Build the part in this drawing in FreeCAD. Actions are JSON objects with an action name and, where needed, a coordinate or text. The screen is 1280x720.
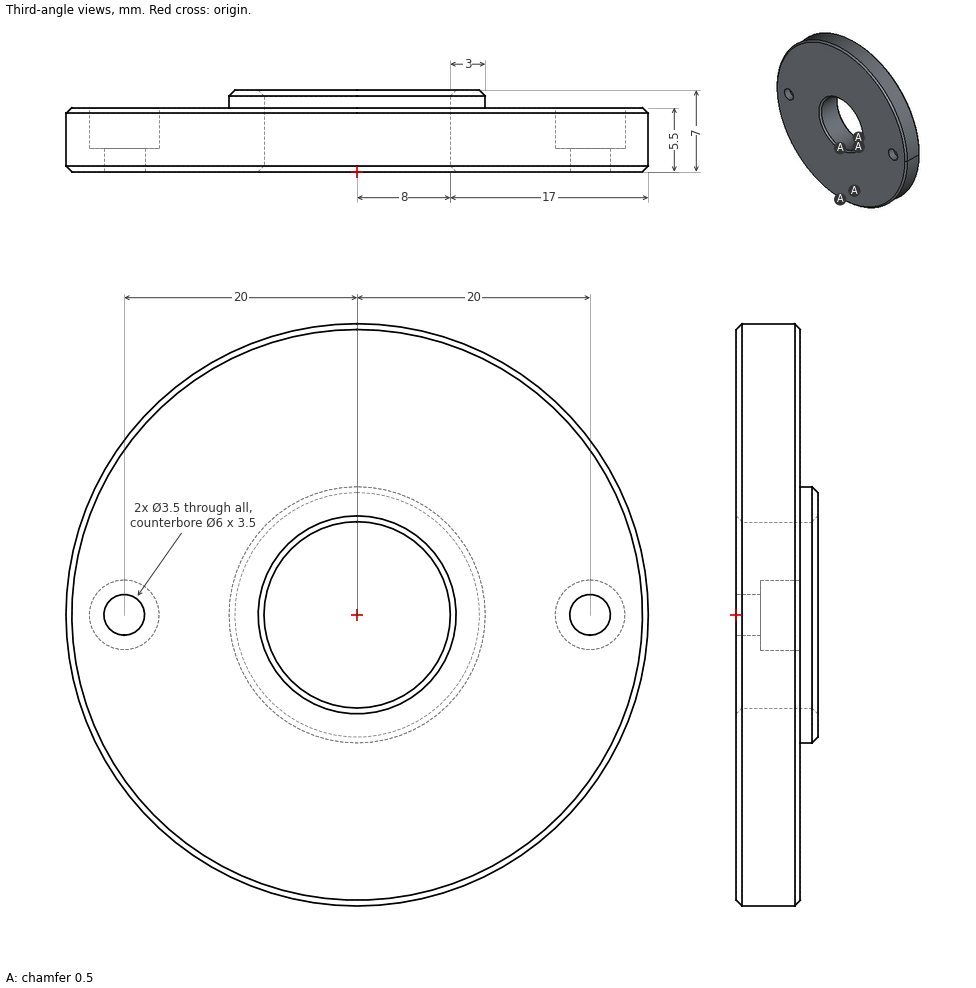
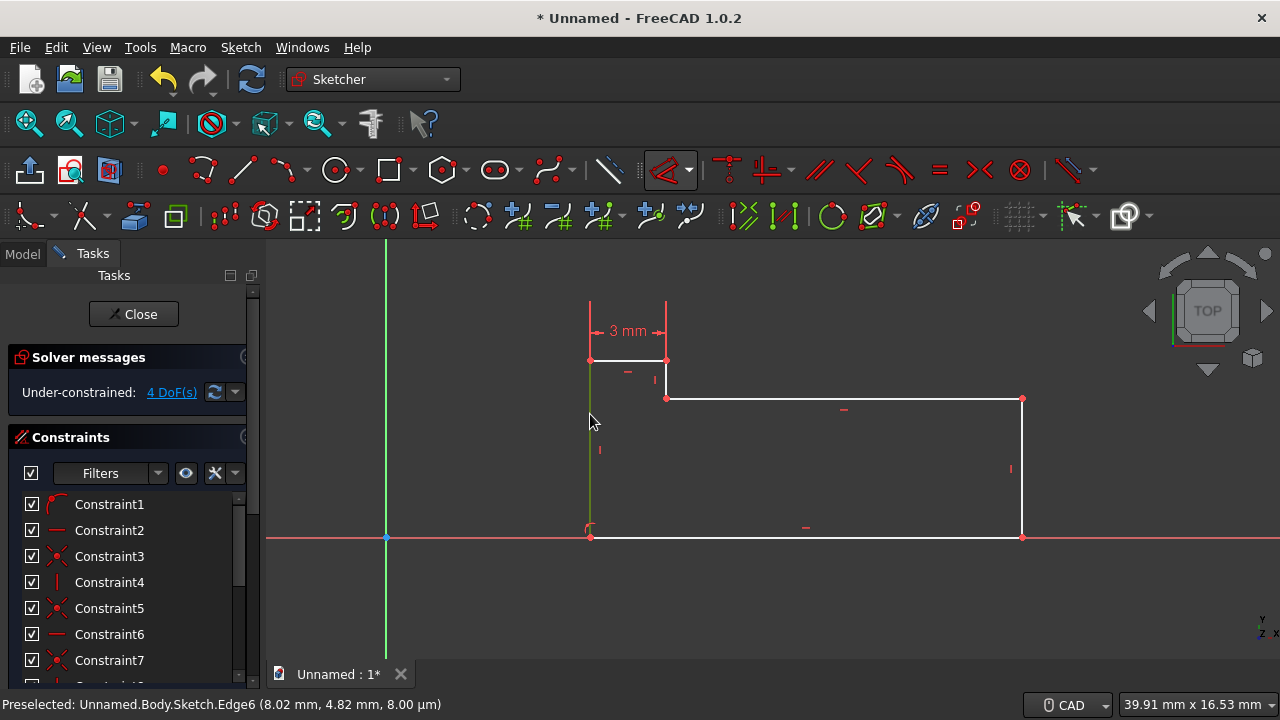
{"action": "left_click", "coordinate": [692, 170]}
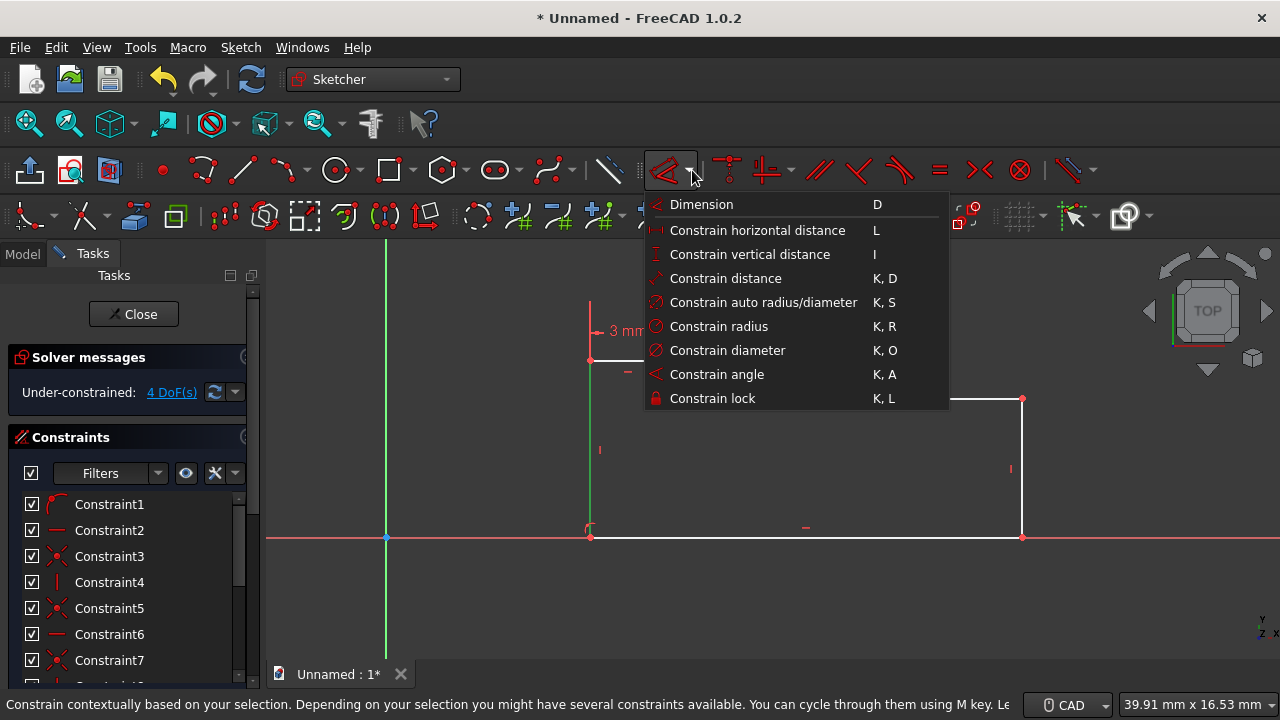
{"action": "left_click", "coordinate": [797, 254]}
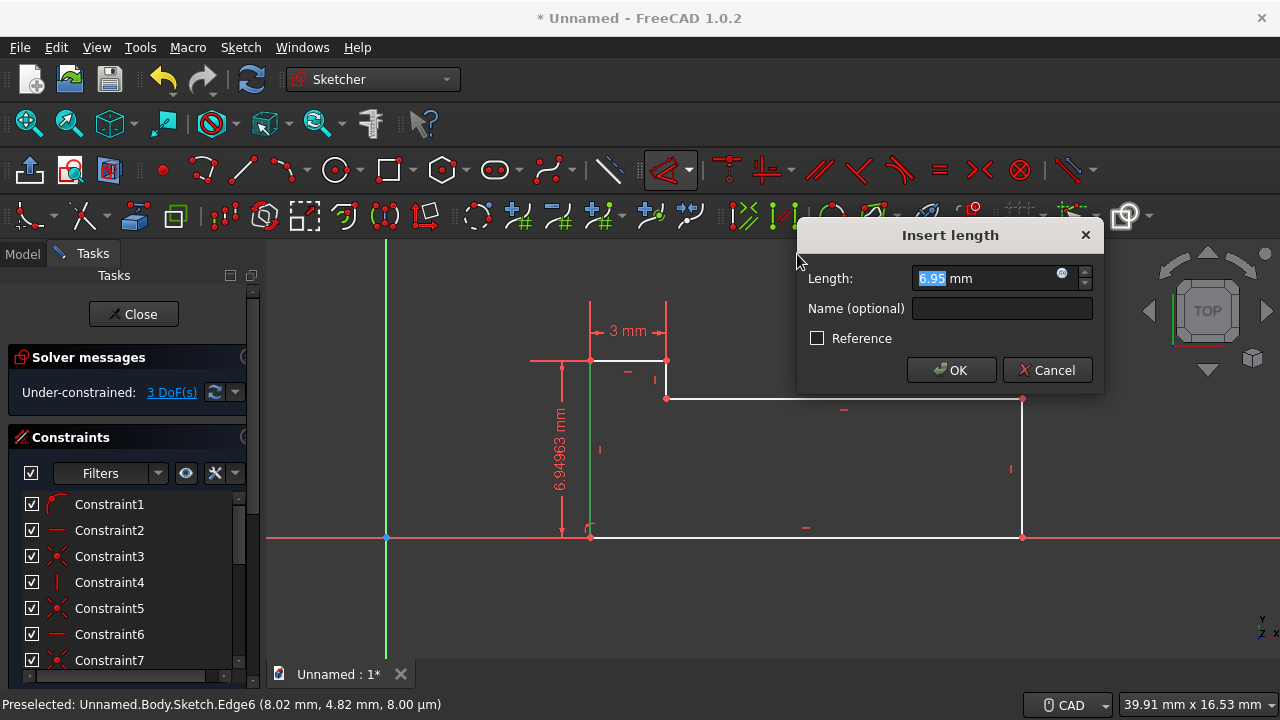
{"action": "type", "text": "7"}
{"action": "key", "text": "Return"}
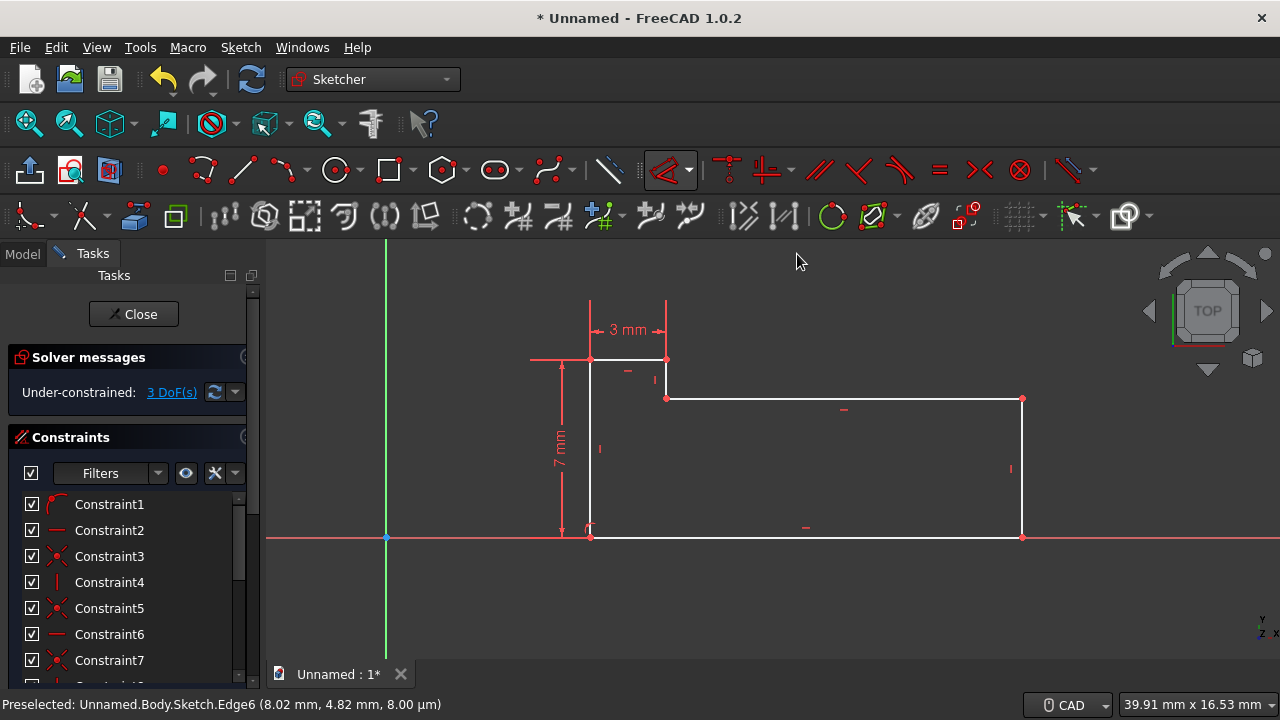
{"action": "left_click", "coordinate": [720, 538]}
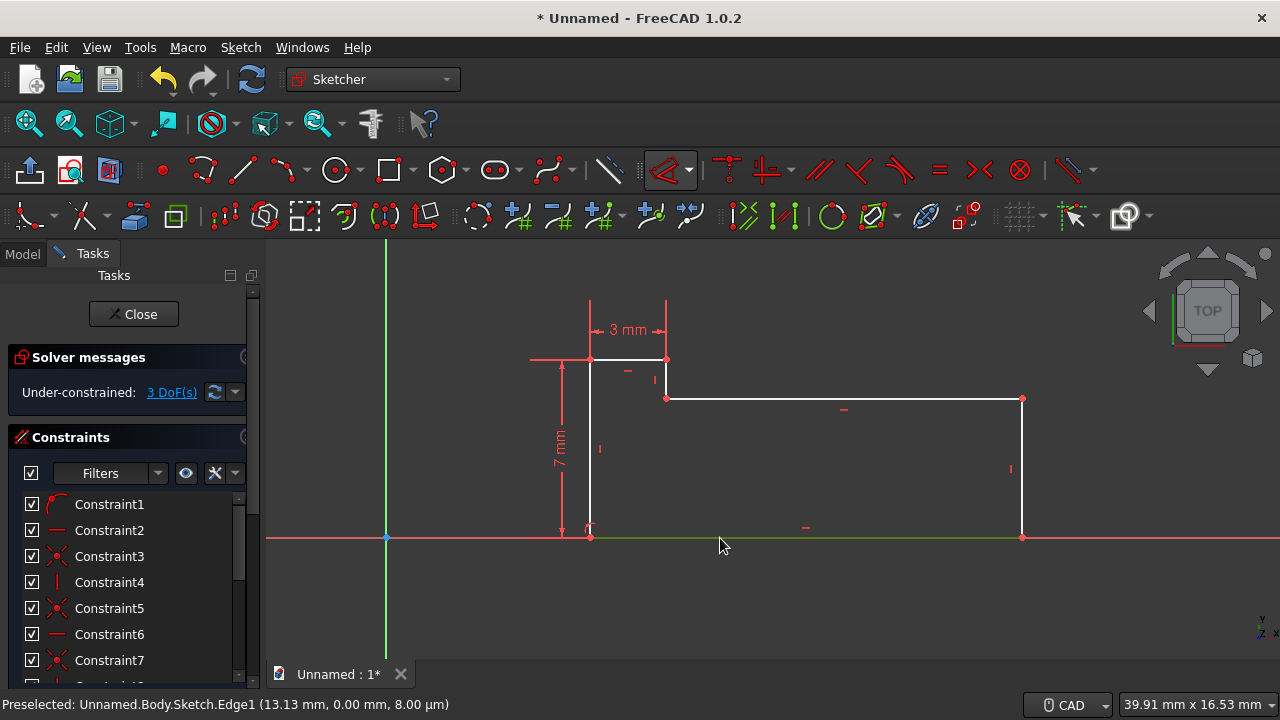
{"action": "left_click", "coordinate": [692, 170]}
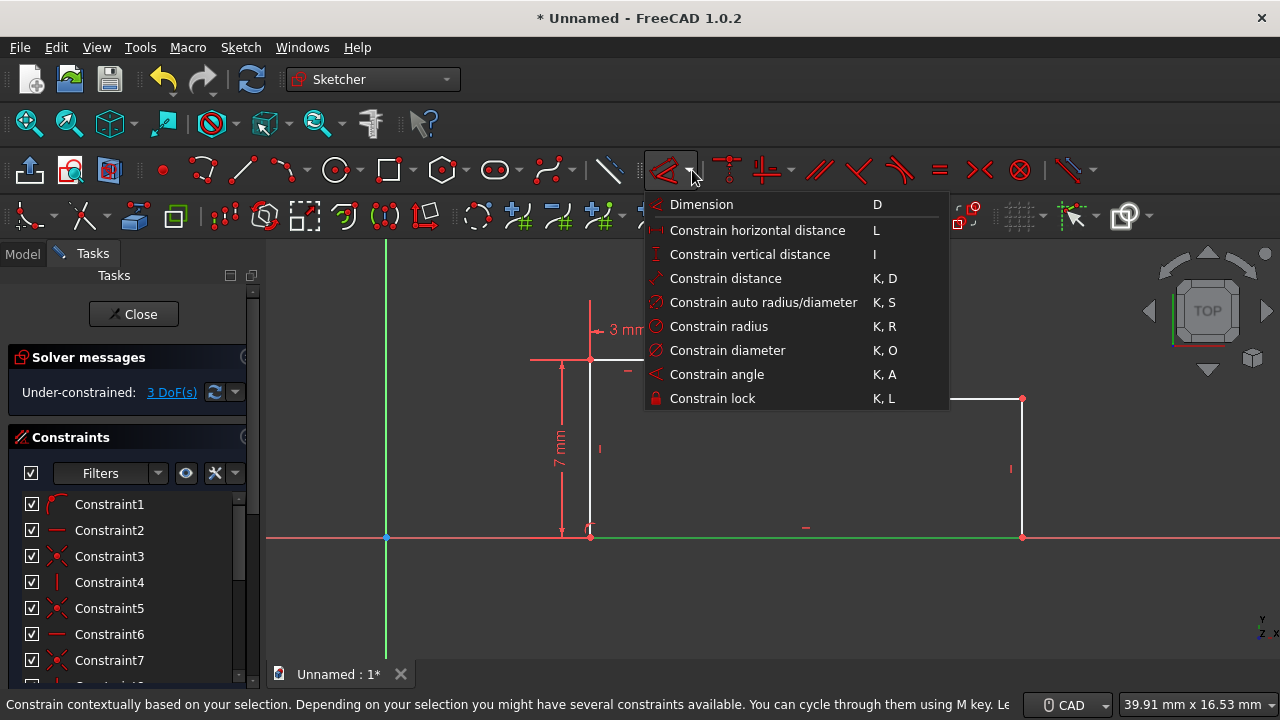
{"action": "left_click", "coordinate": [797, 230]}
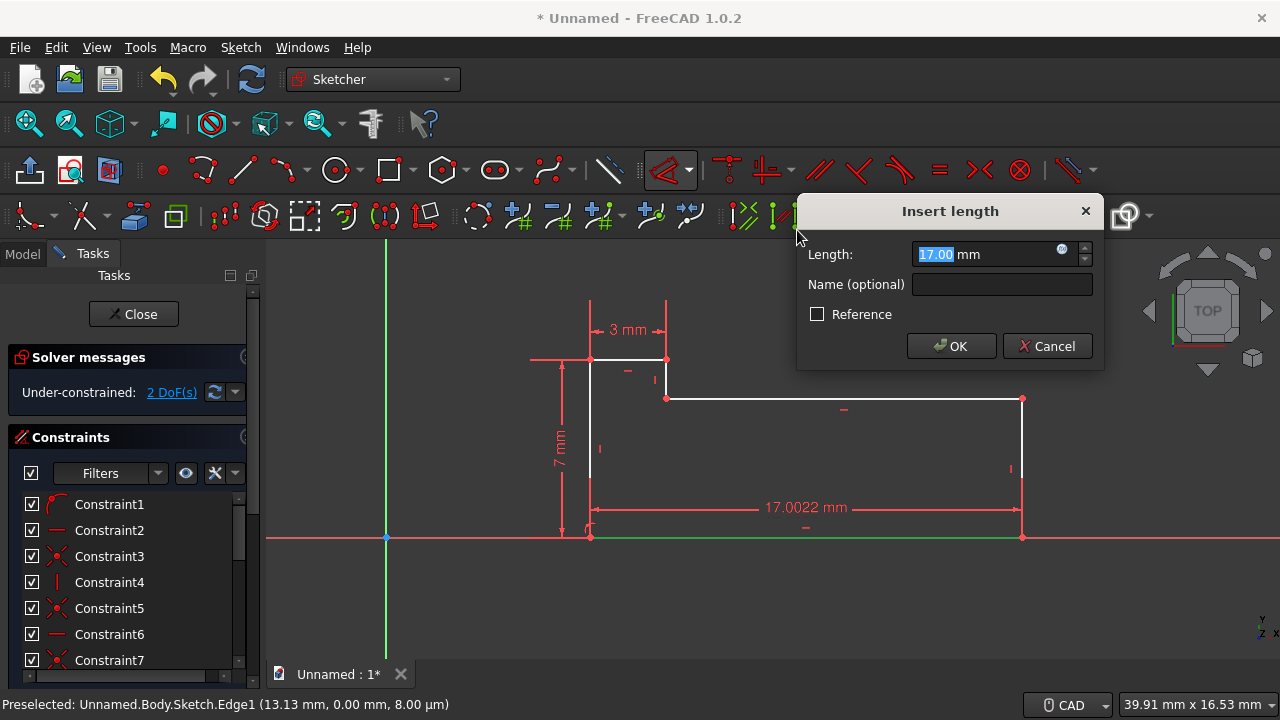
{"action": "type", "text": "17"}
{"action": "key", "text": "Return"}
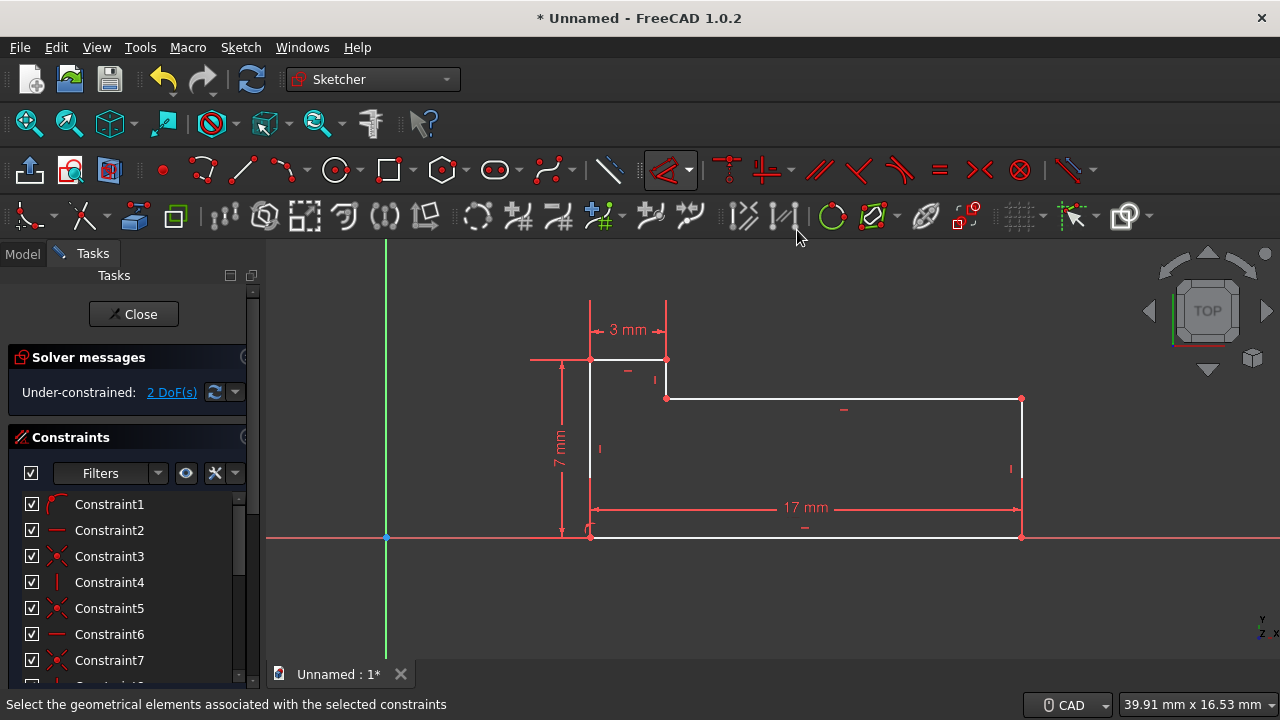
{"action": "left_click", "coordinate": [590, 538]}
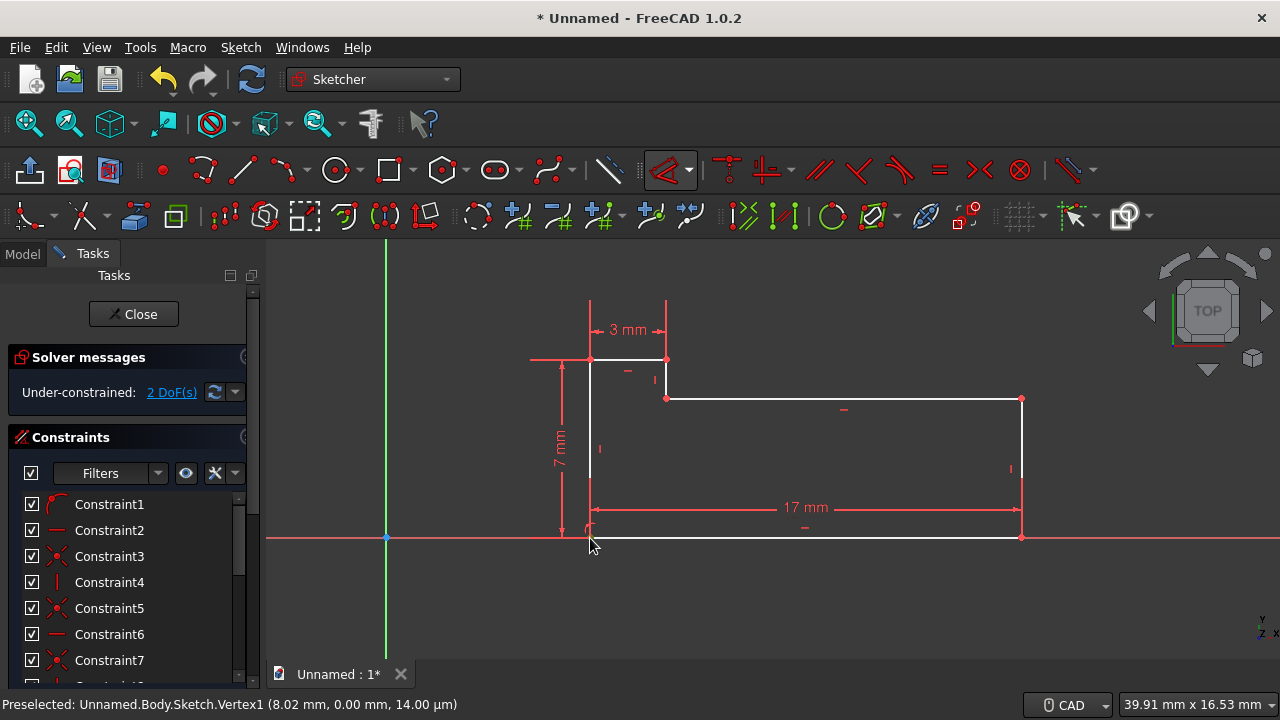
{"action": "key", "text": "l"}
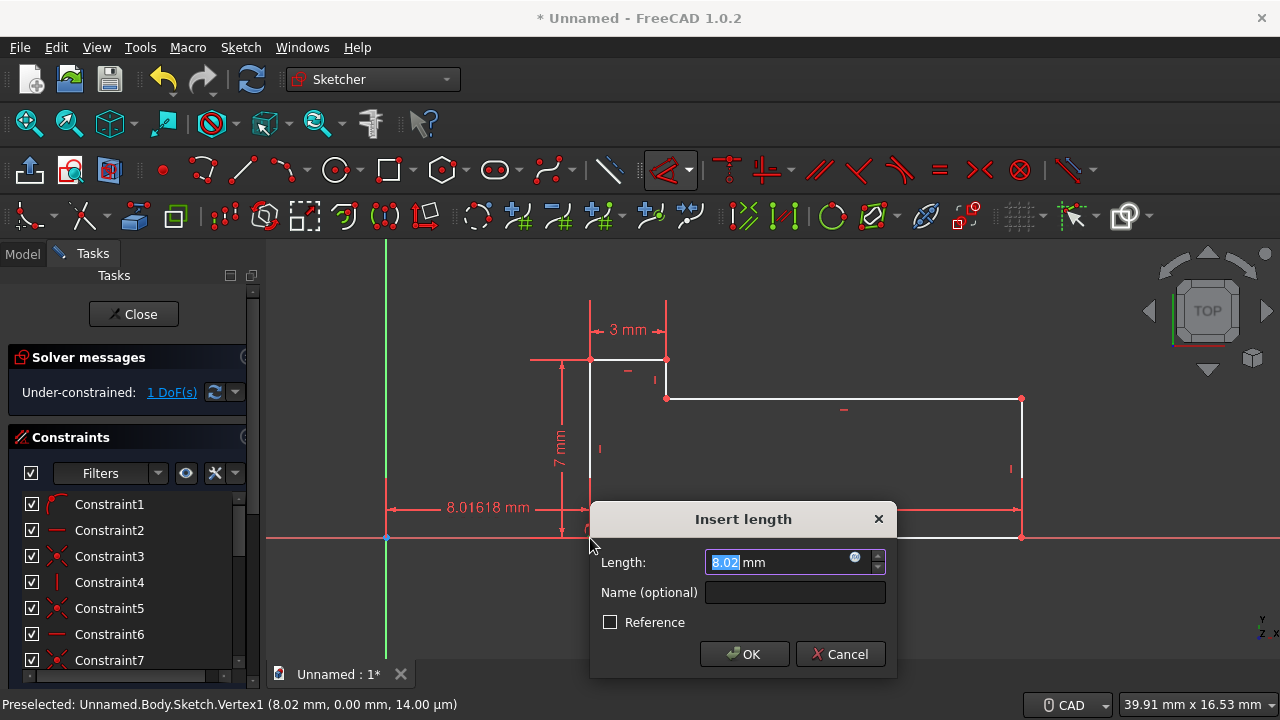
{"action": "type", "text": "8"}
{"action": "key", "text": "Return"}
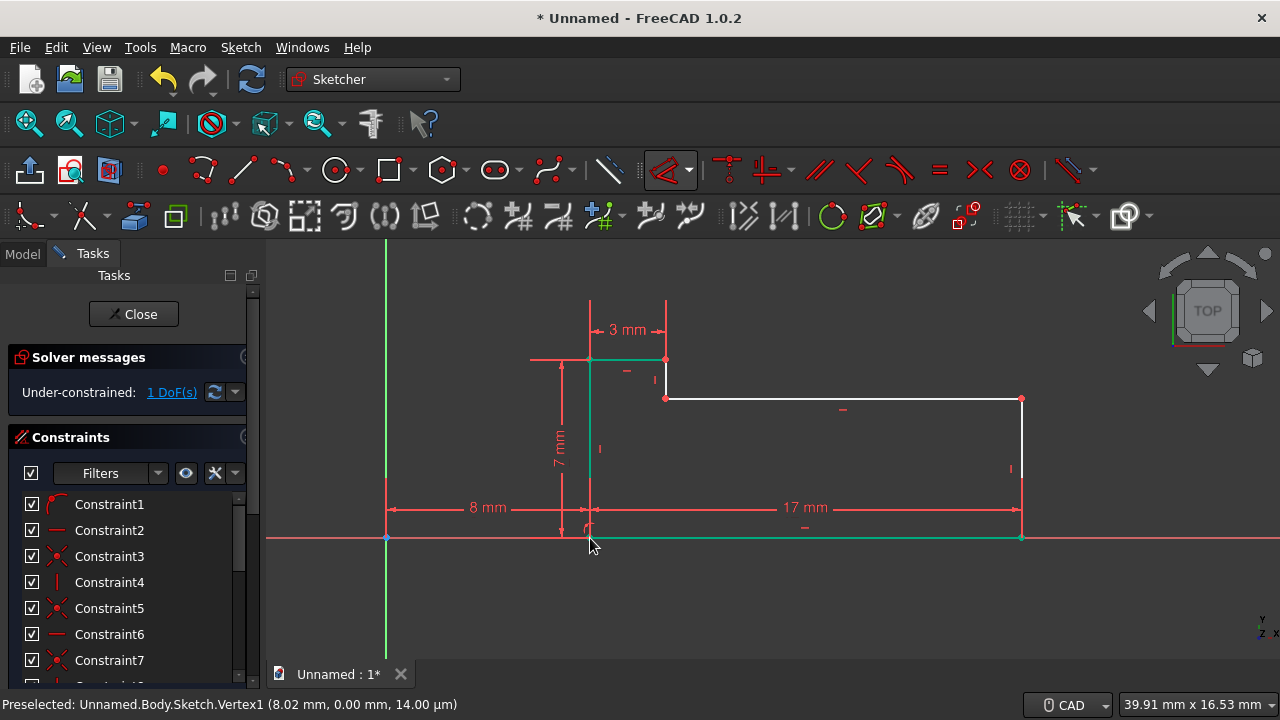
{"action": "left_click", "coordinate": [1022, 496]}